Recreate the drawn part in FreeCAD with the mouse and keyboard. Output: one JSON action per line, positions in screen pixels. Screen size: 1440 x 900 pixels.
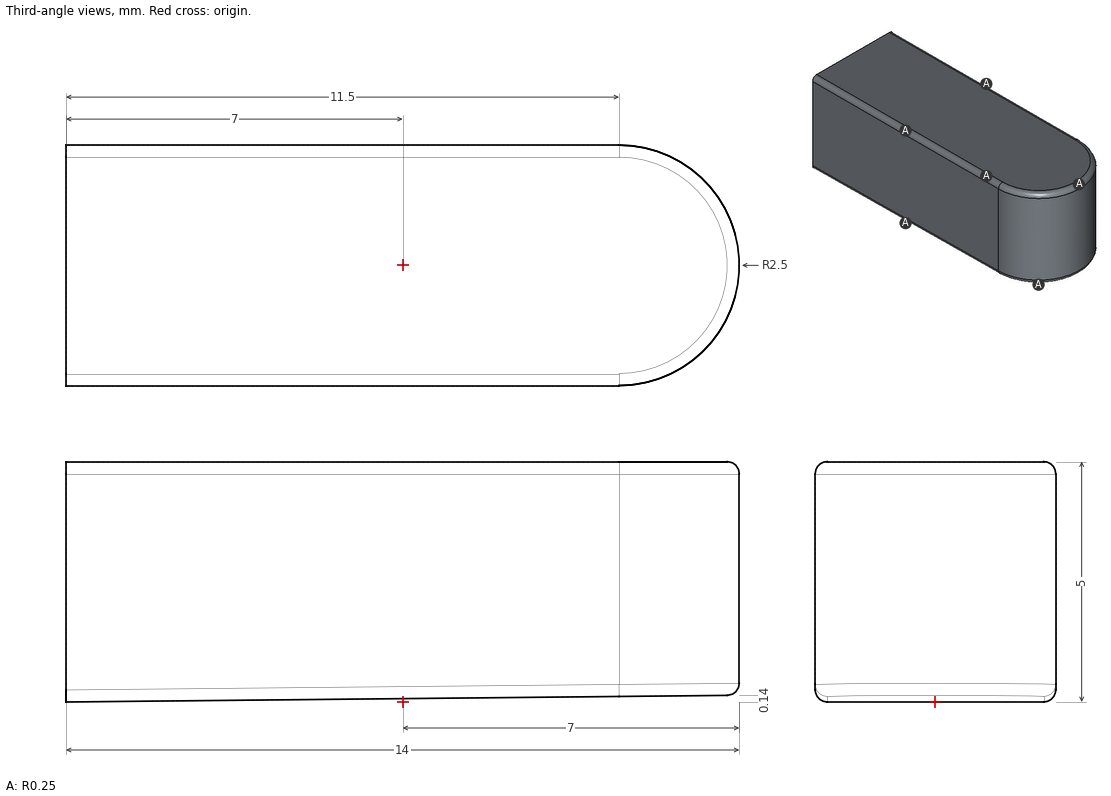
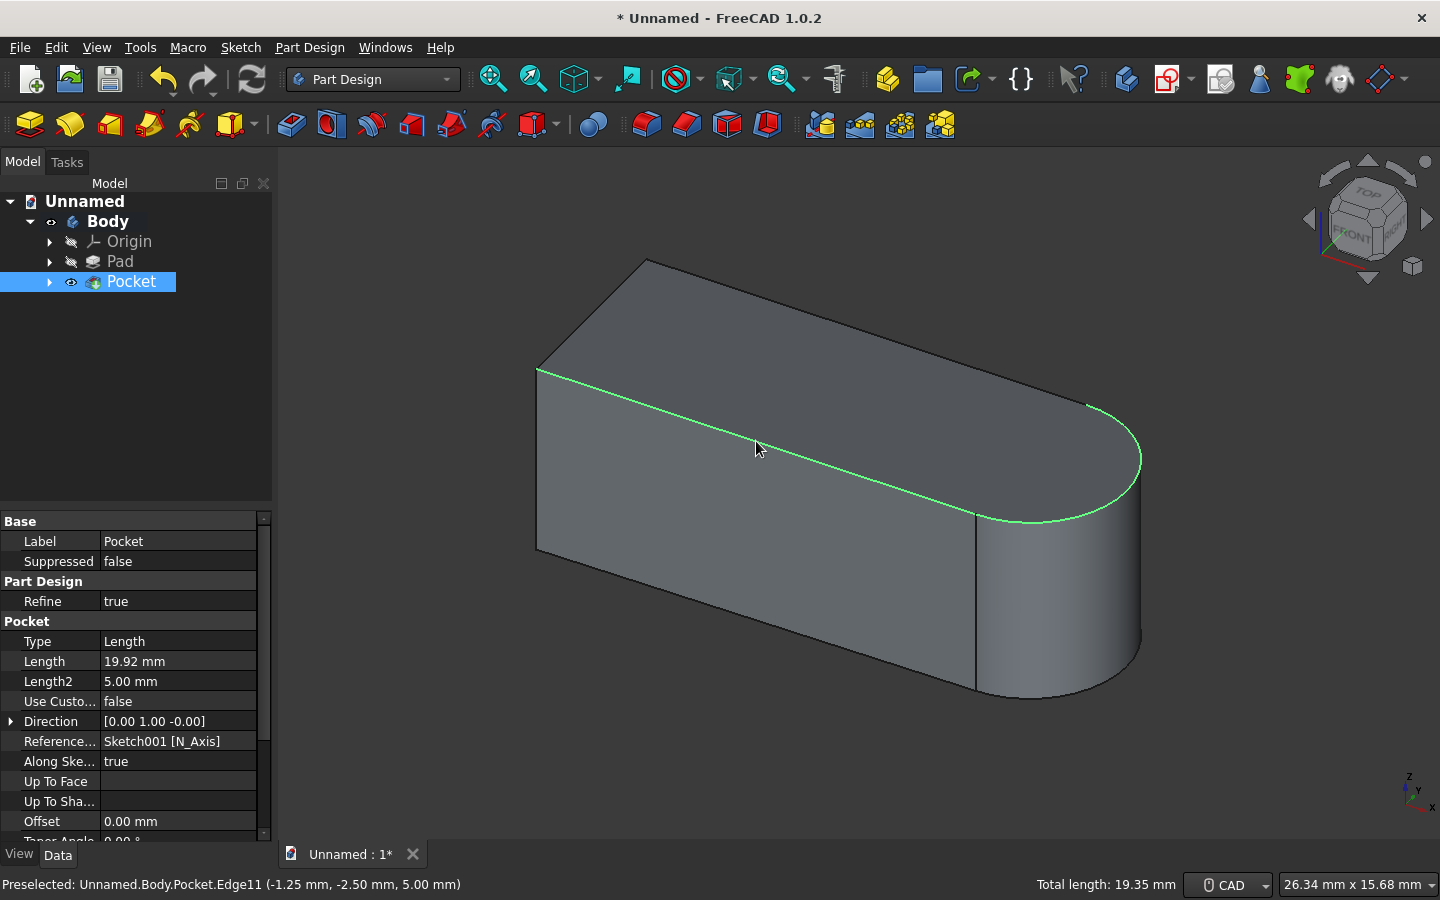
{"action": "key", "text": "0"}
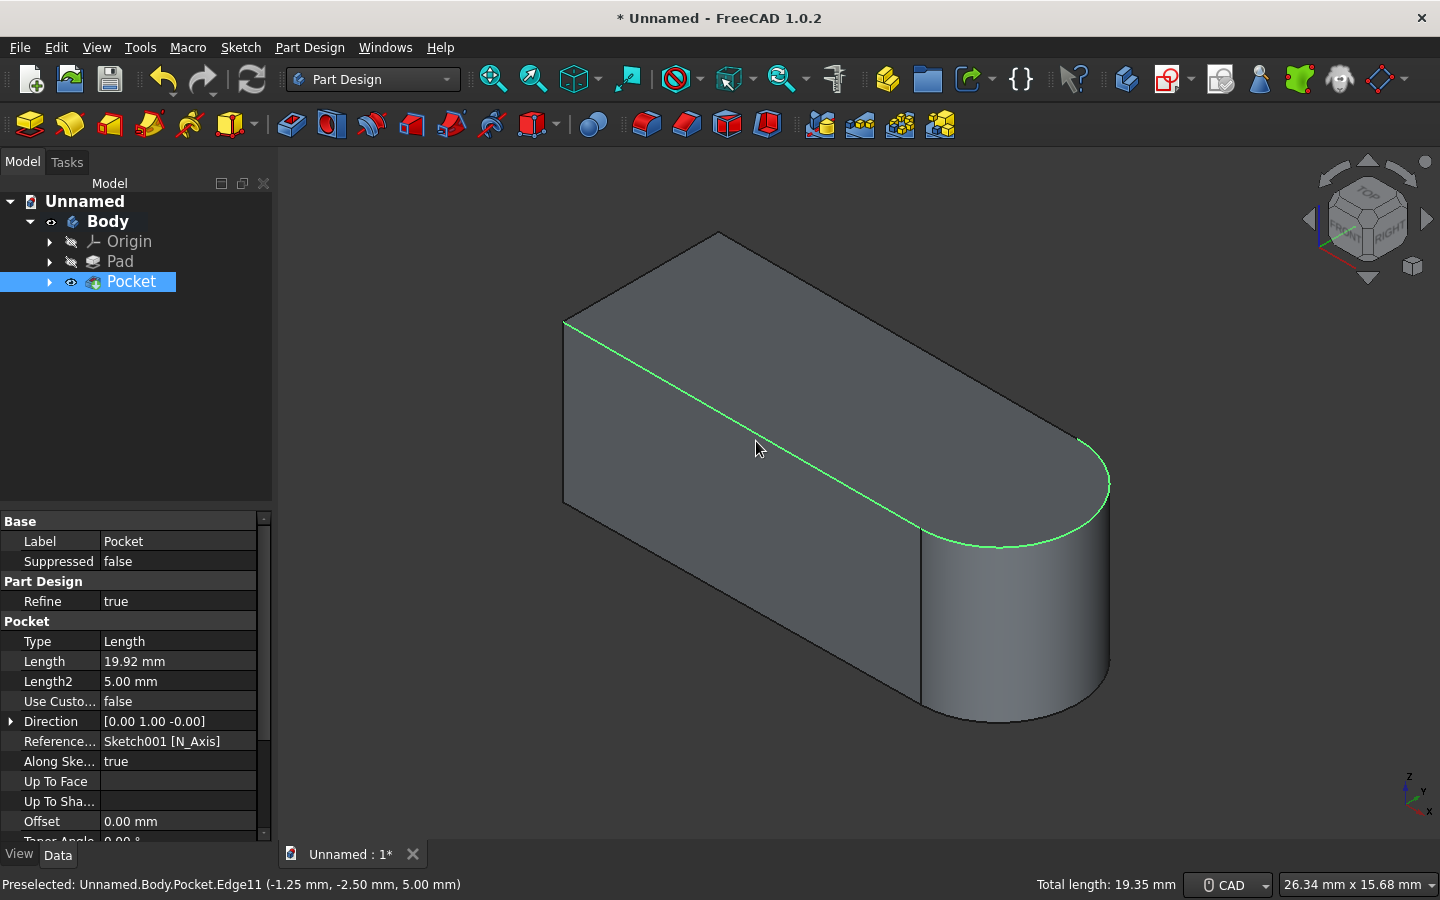
{"action": "key", "text": "2"}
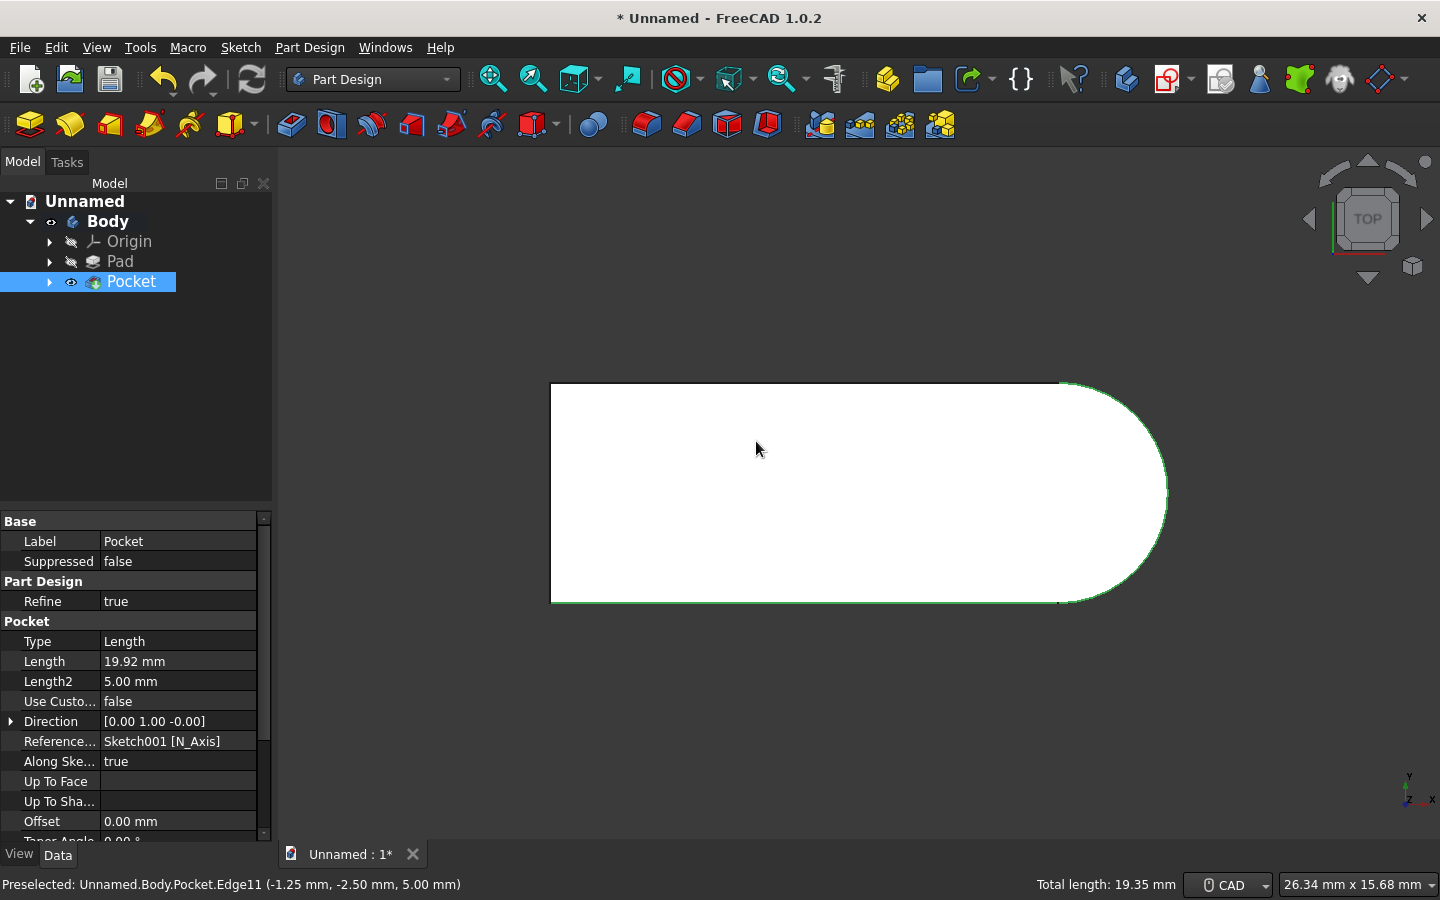
{"action": "left_click", "coordinate": [804, 382], "text": "ctrl"}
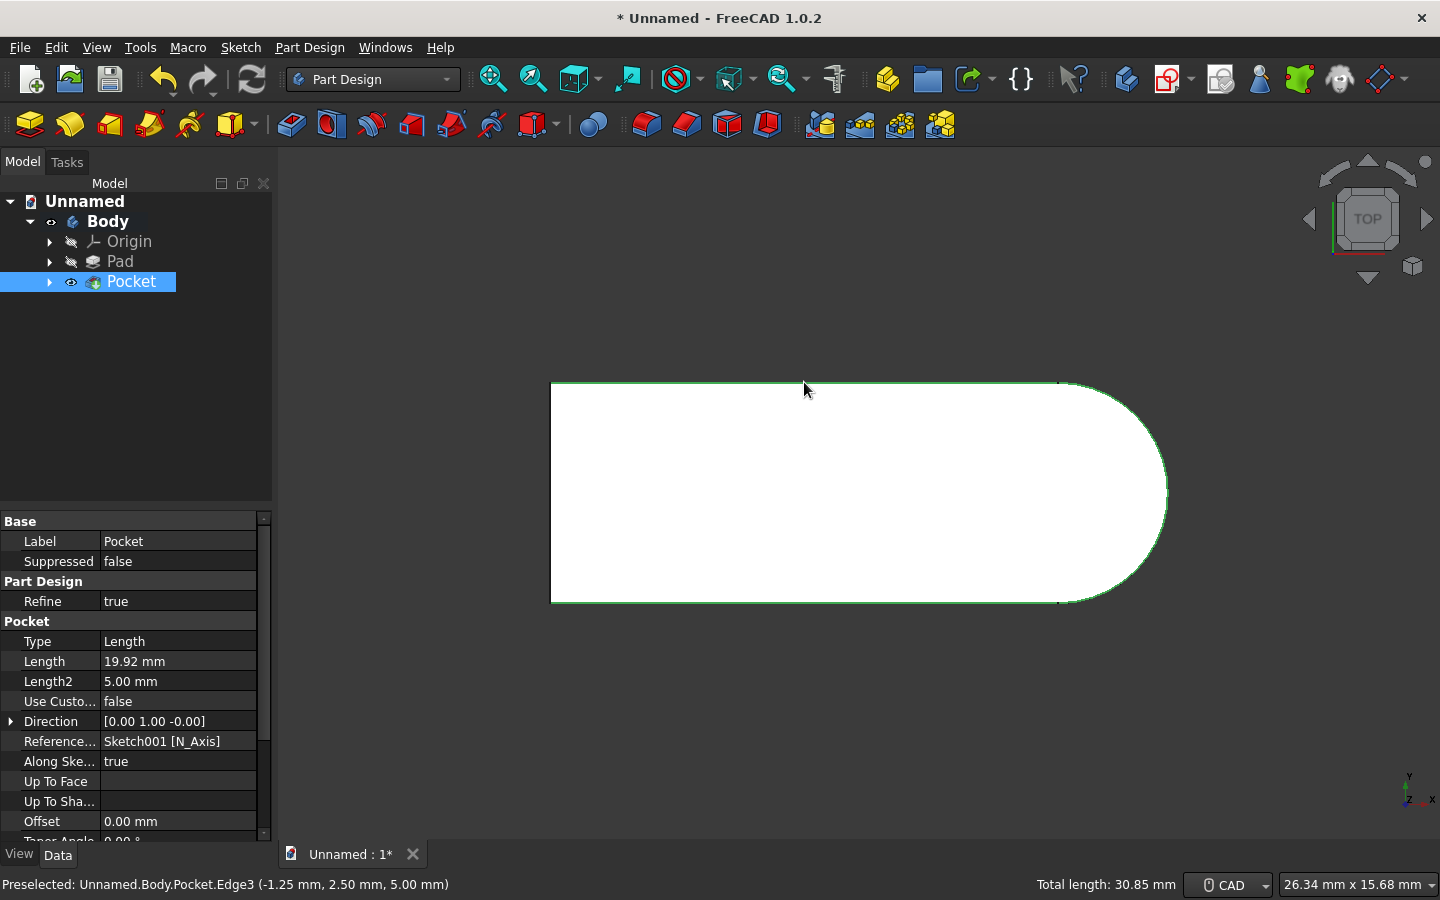
{"action": "key", "text": "1"}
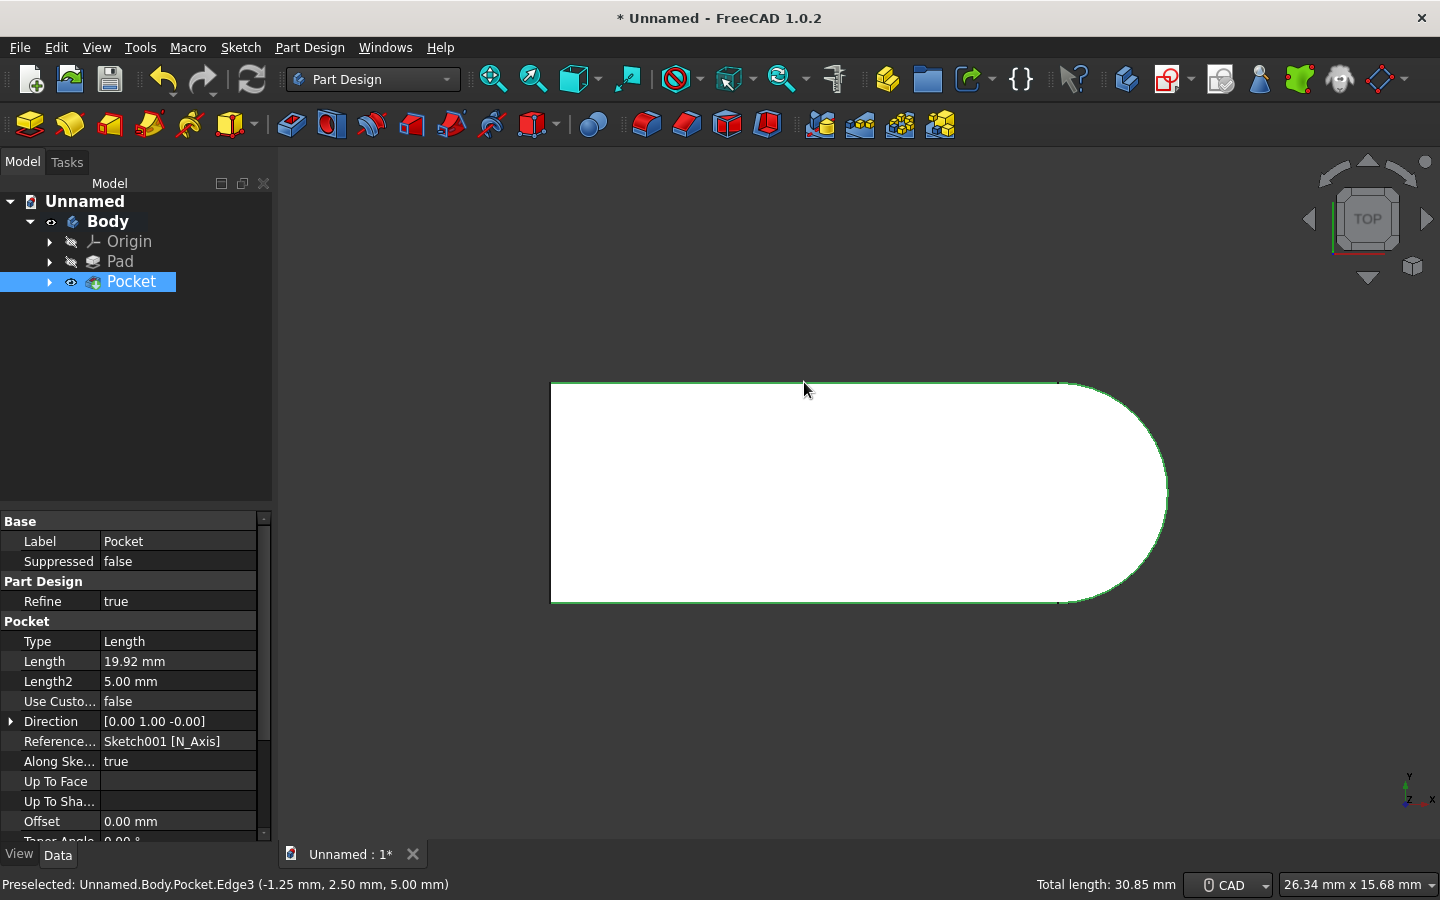
{"action": "left_click", "coordinate": [804, 600], "text": "ctrl"}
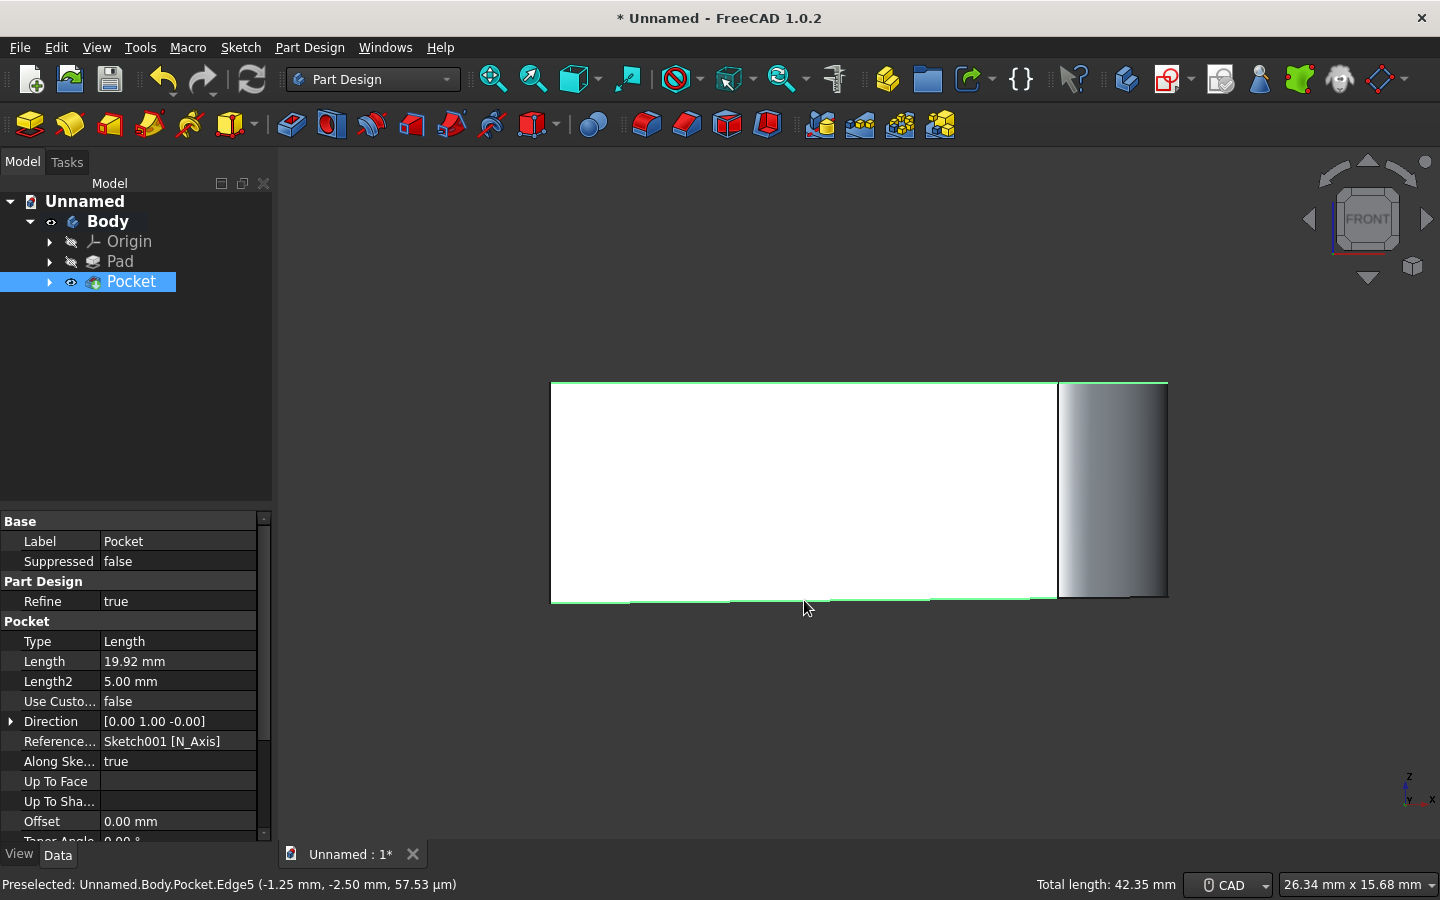
{"action": "left_click", "coordinate": [1136, 596], "text": "ctrl"}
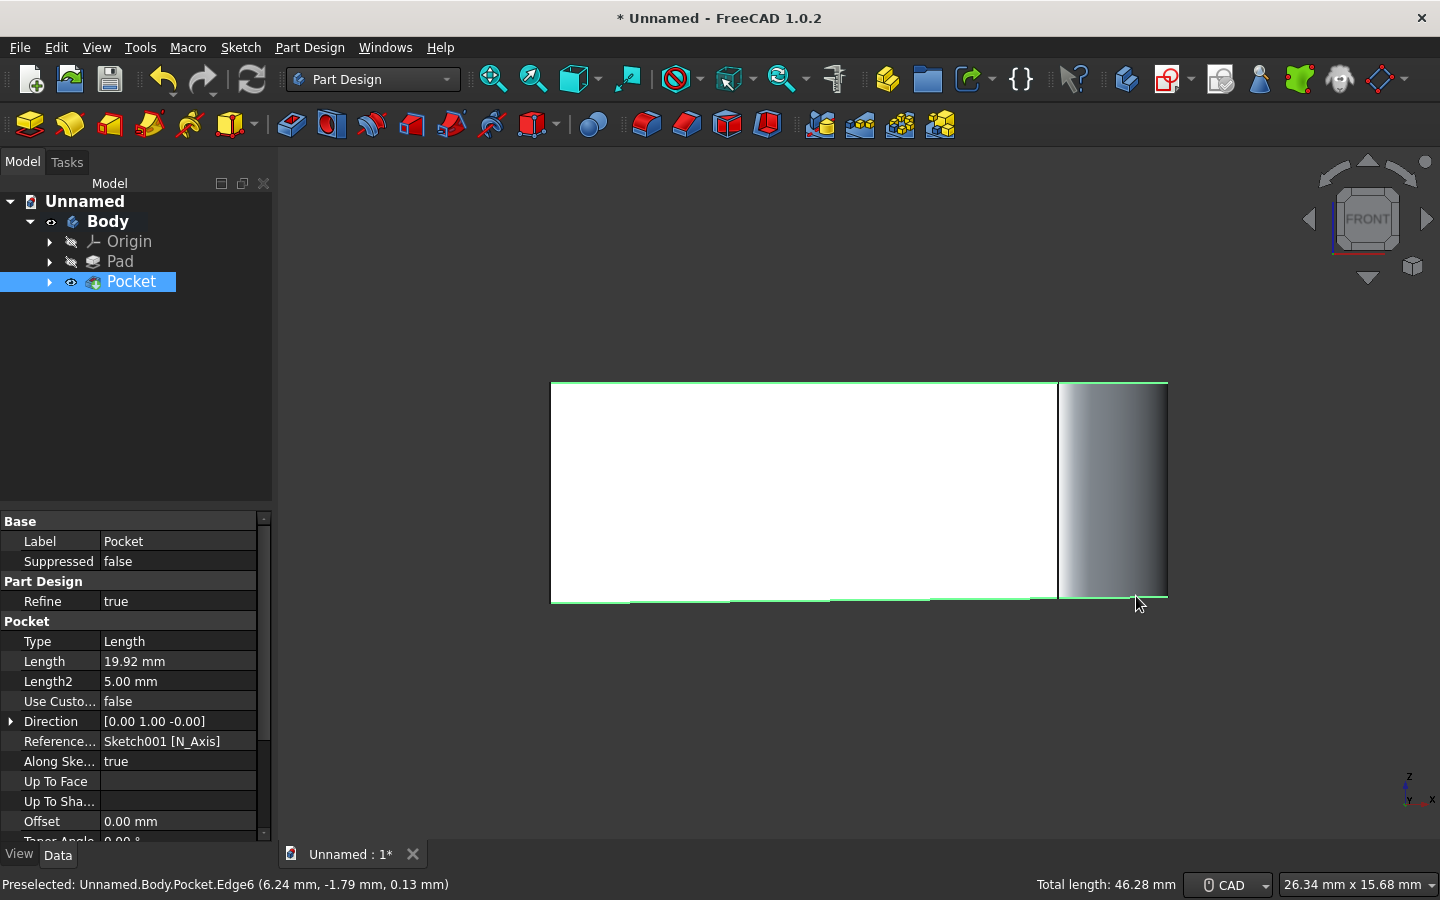
{"action": "key", "text": "3"}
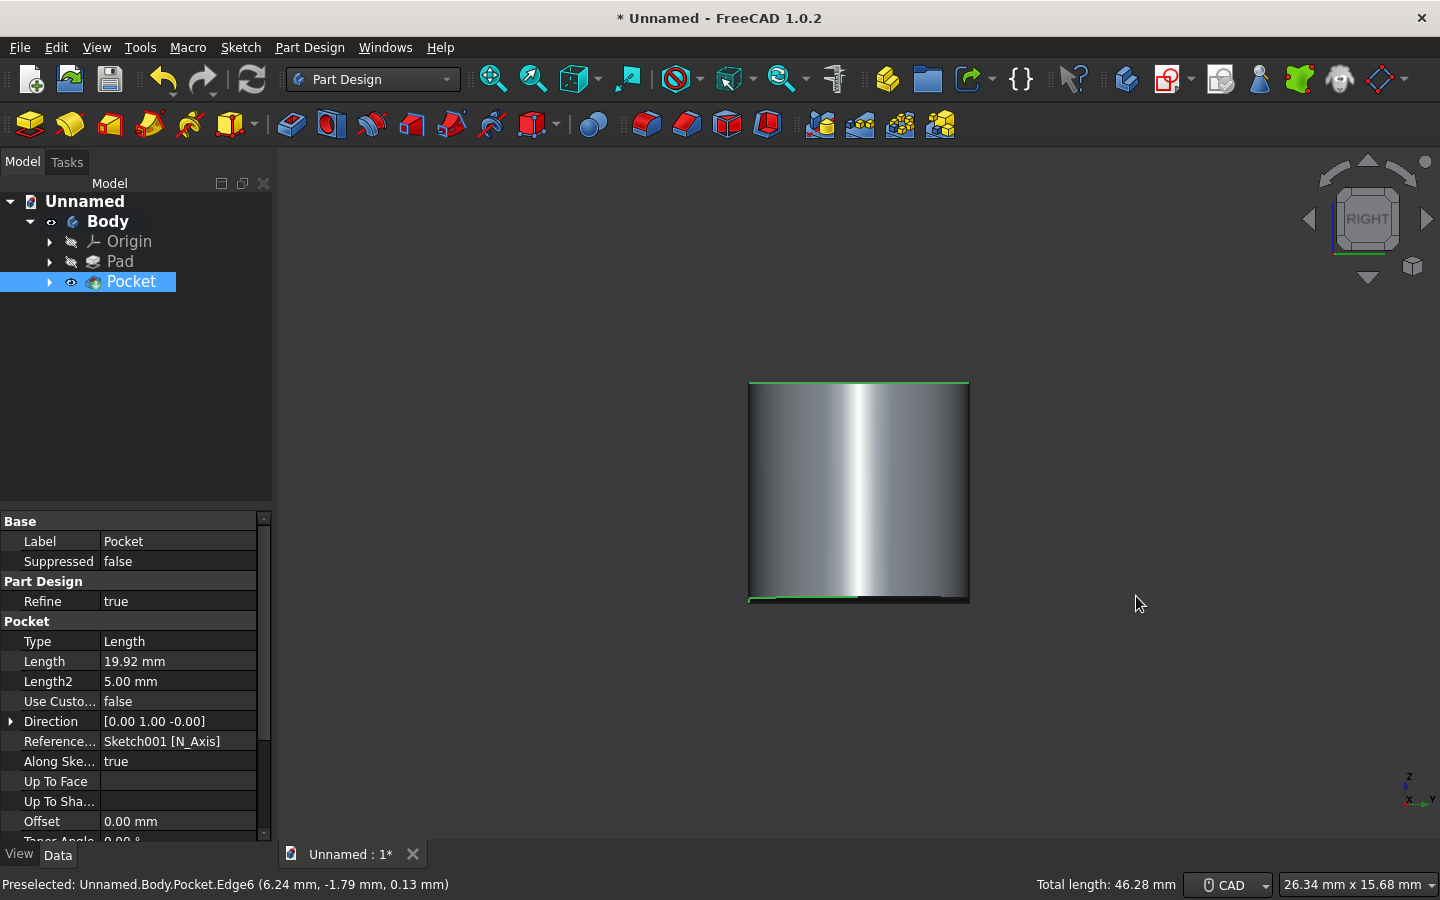
{"action": "left_click", "coordinate": [494, 80]}